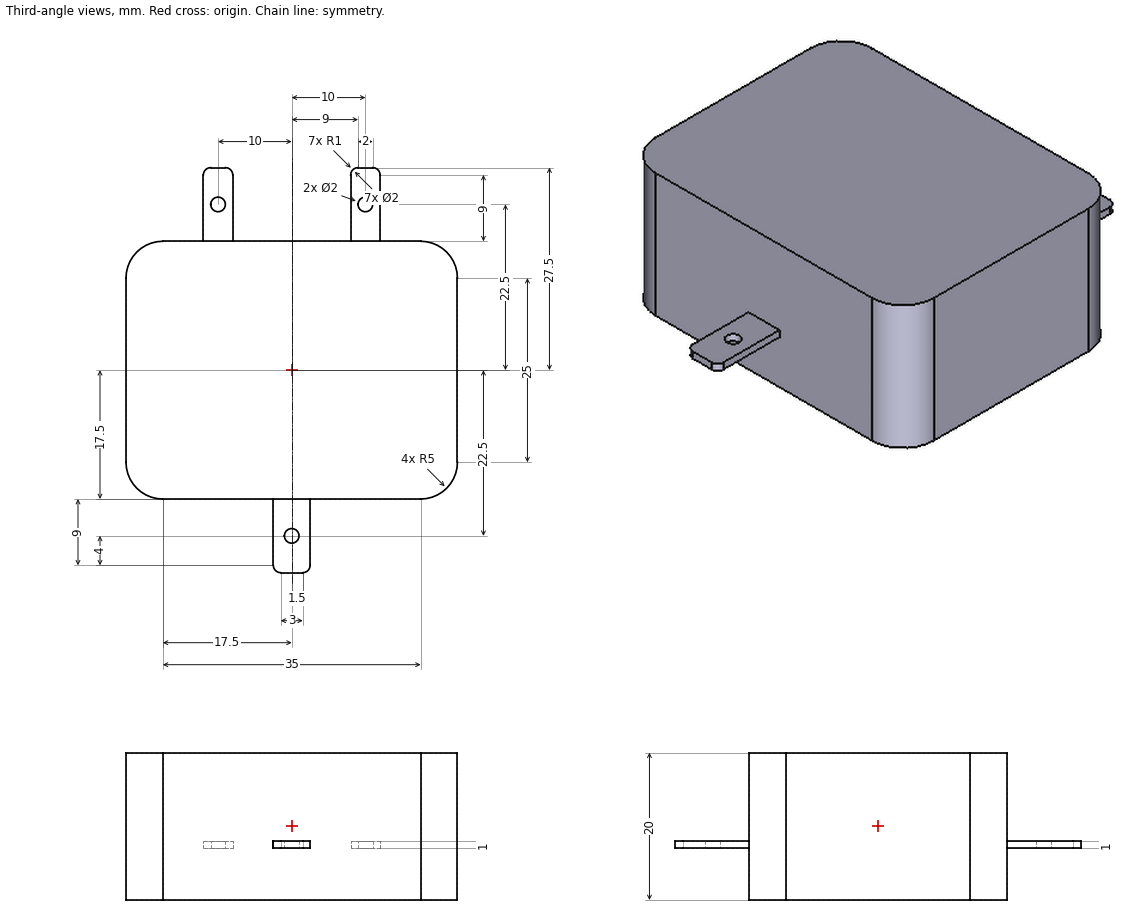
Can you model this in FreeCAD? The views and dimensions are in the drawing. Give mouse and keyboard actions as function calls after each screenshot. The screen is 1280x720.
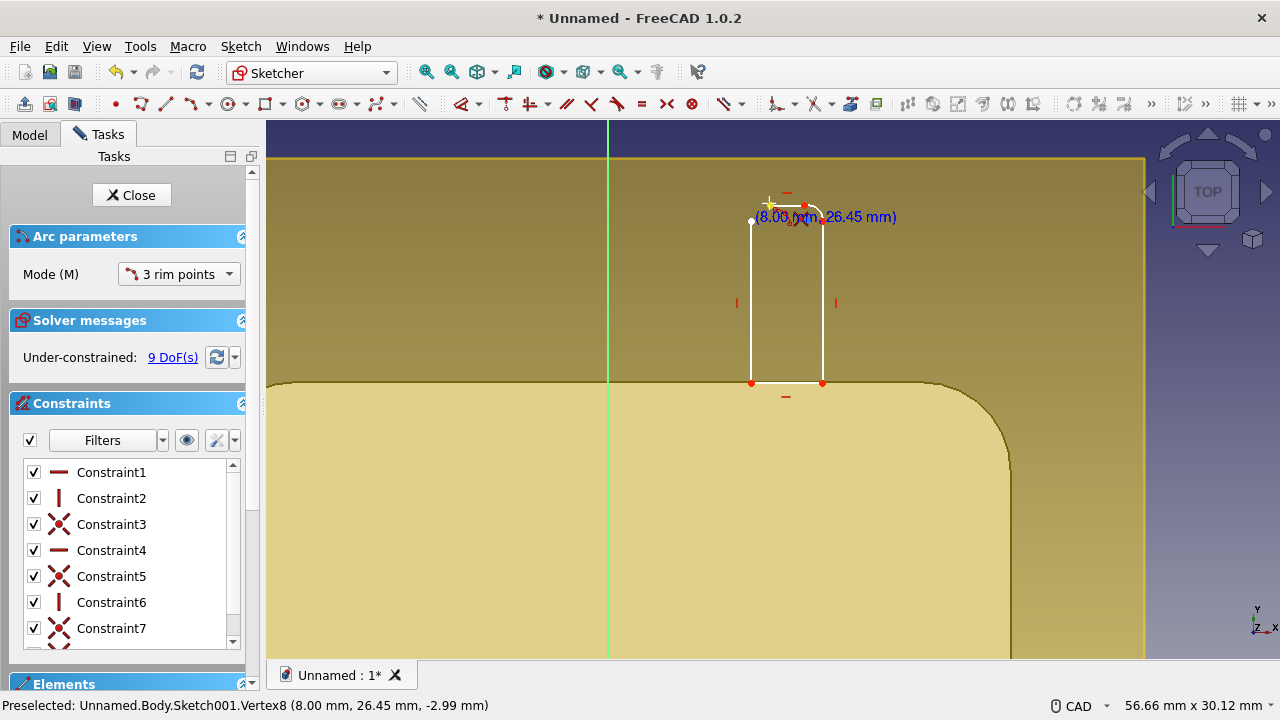
click(771, 206)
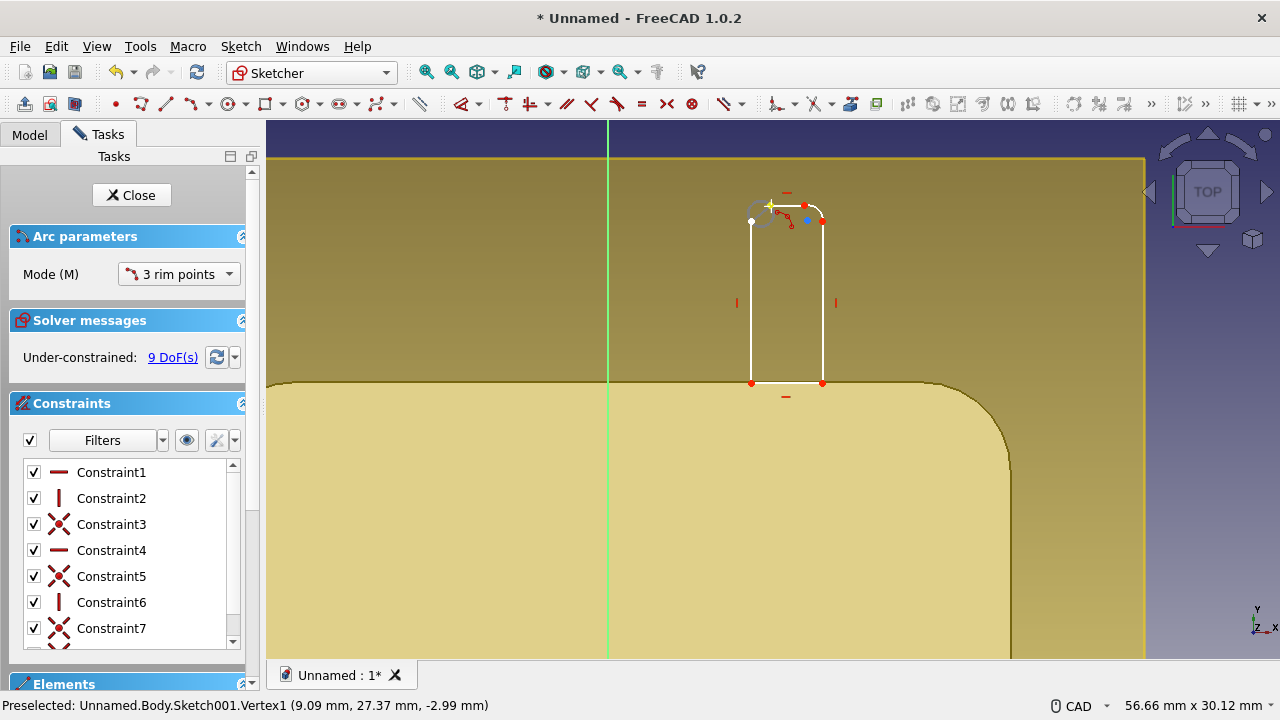
scroll(756, 208, up, 6)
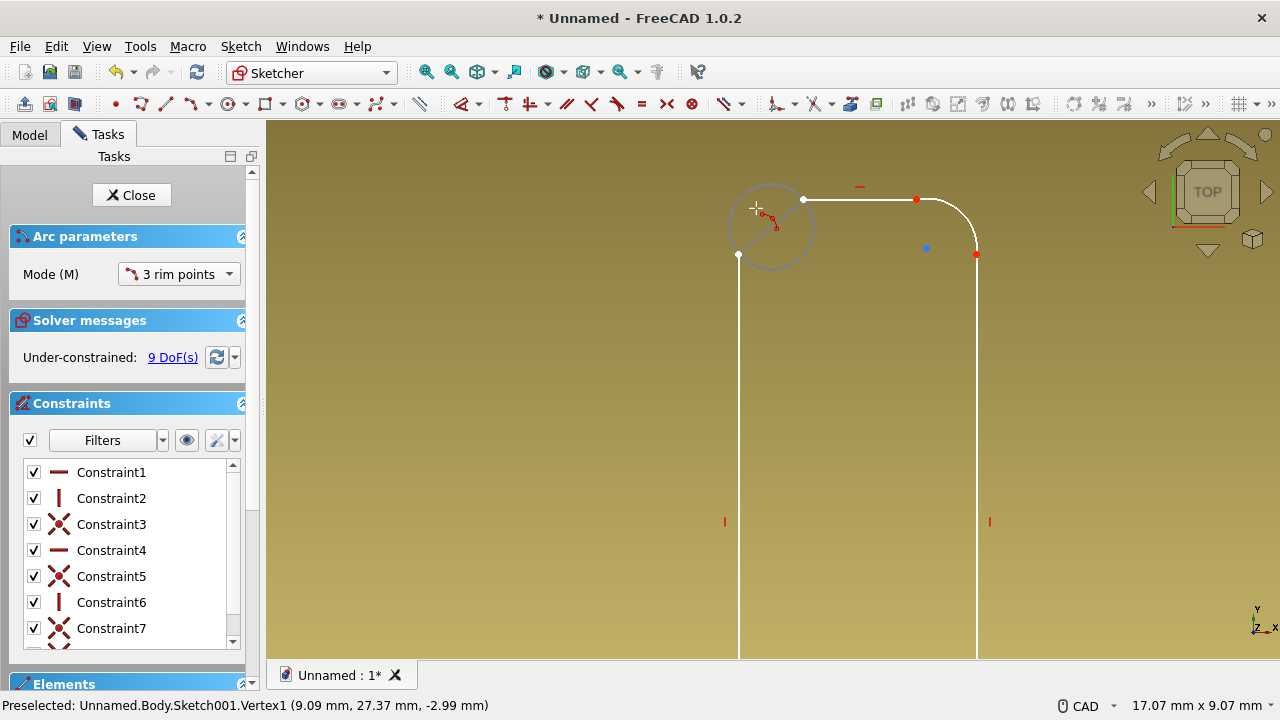
click(756, 209)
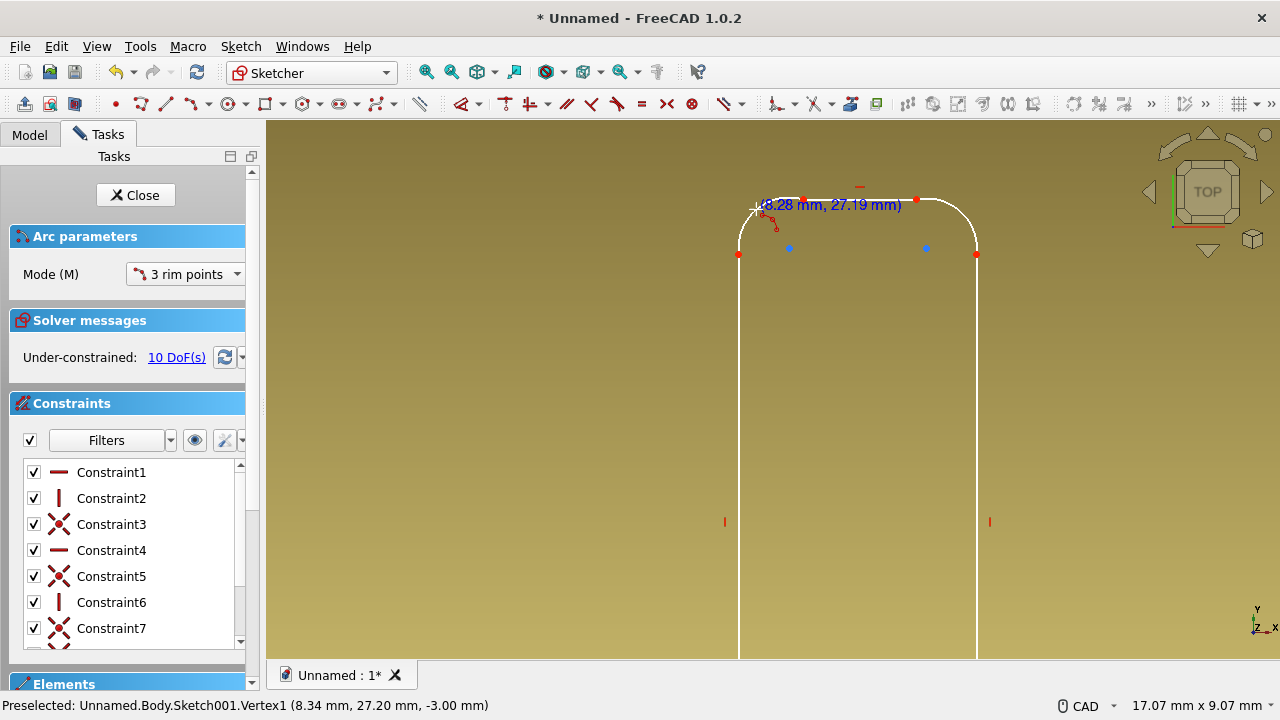
key(g)
key(l)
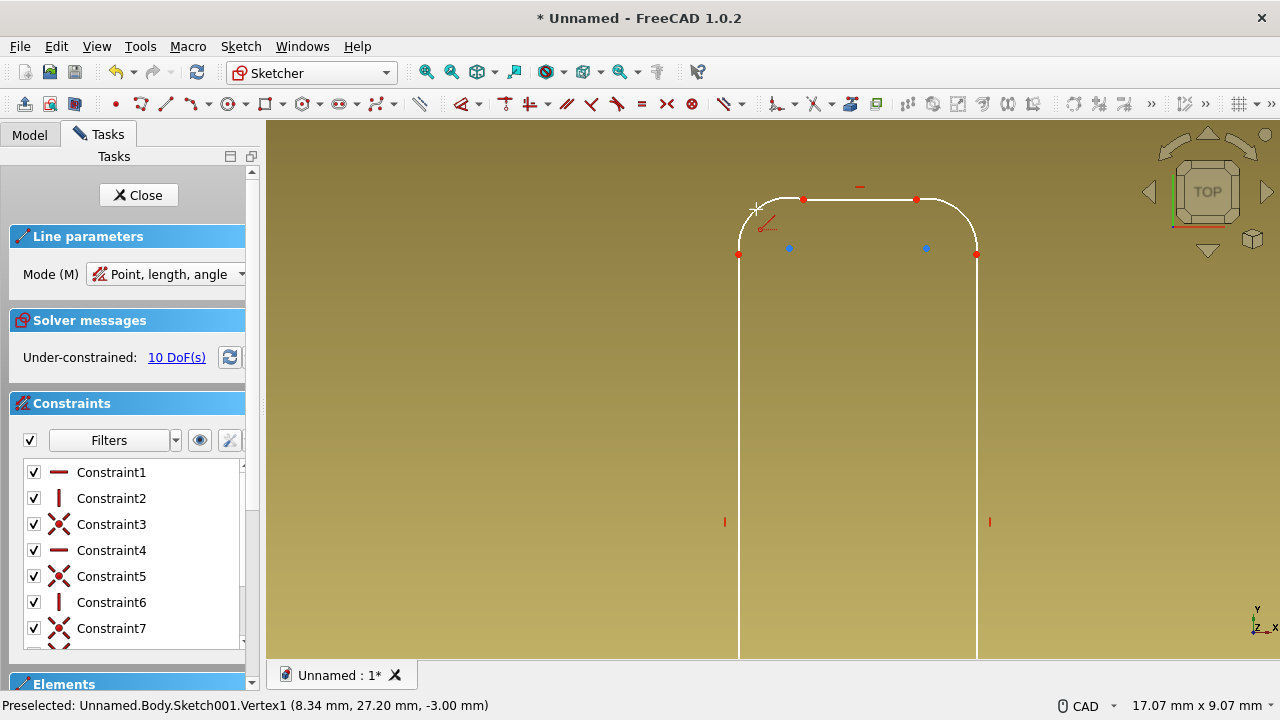
scroll(759, 211, down, 11)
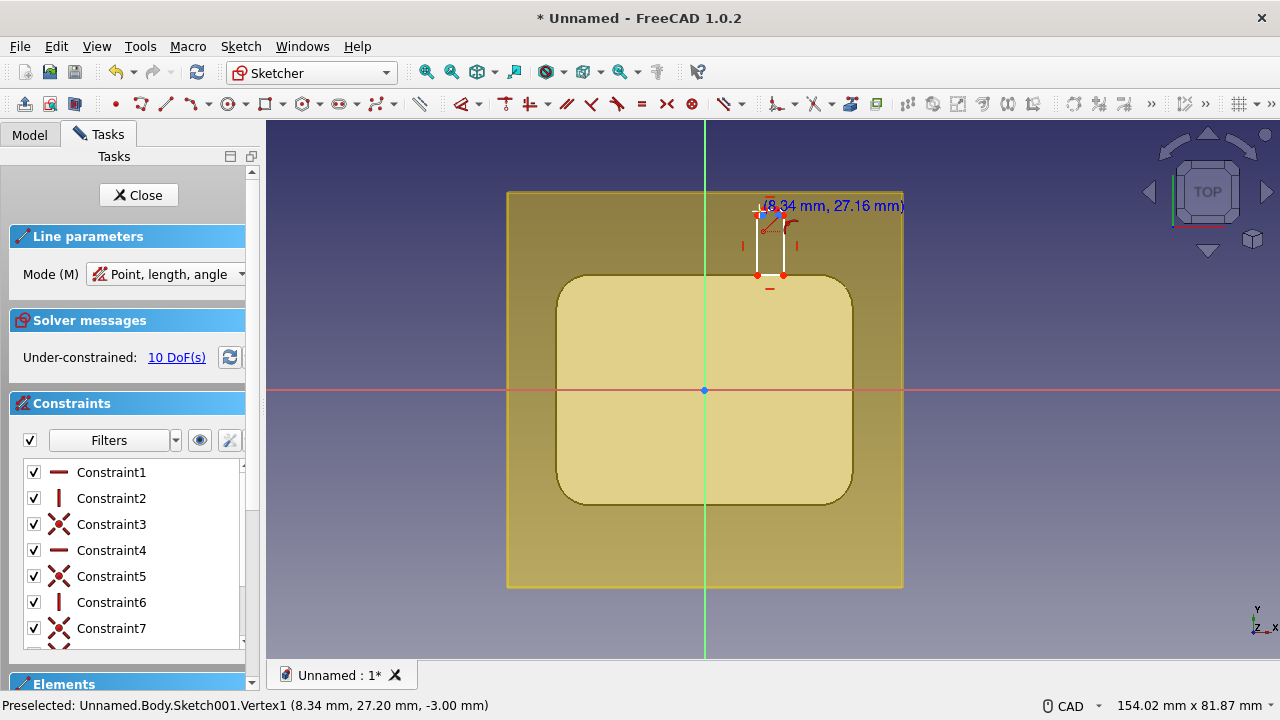
click(632, 209)
click(645, 209)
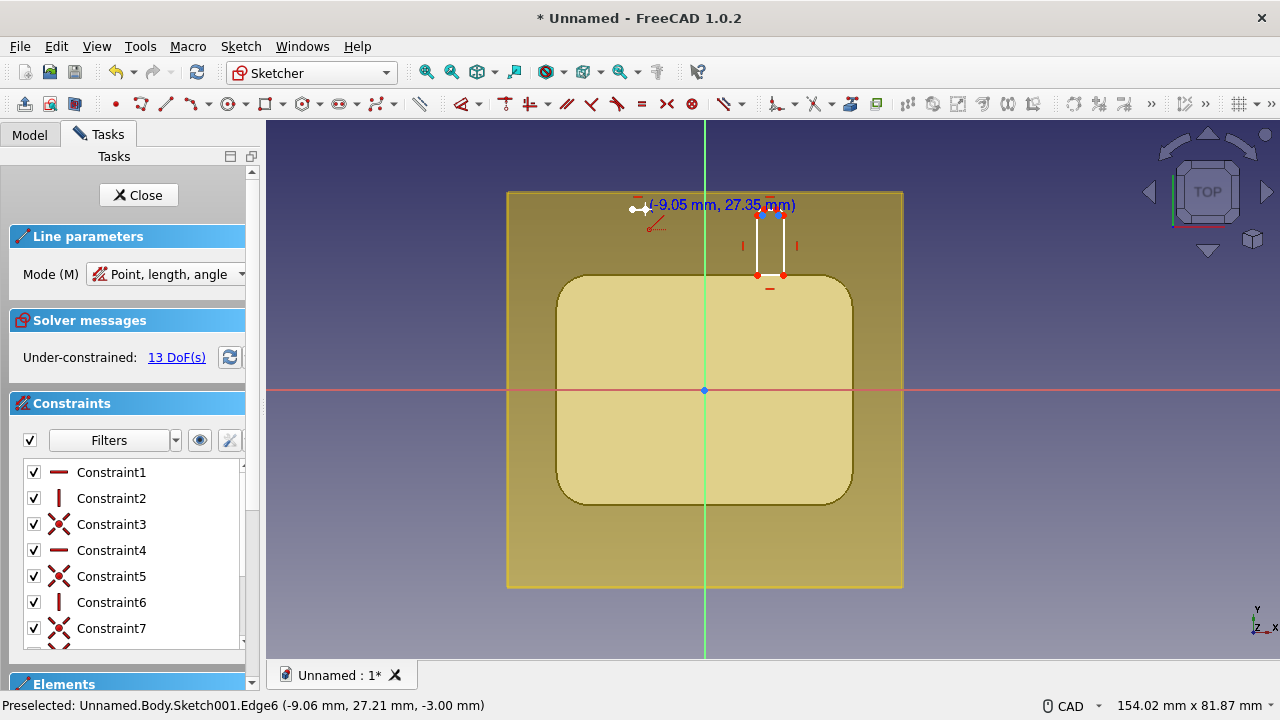
click(141, 104)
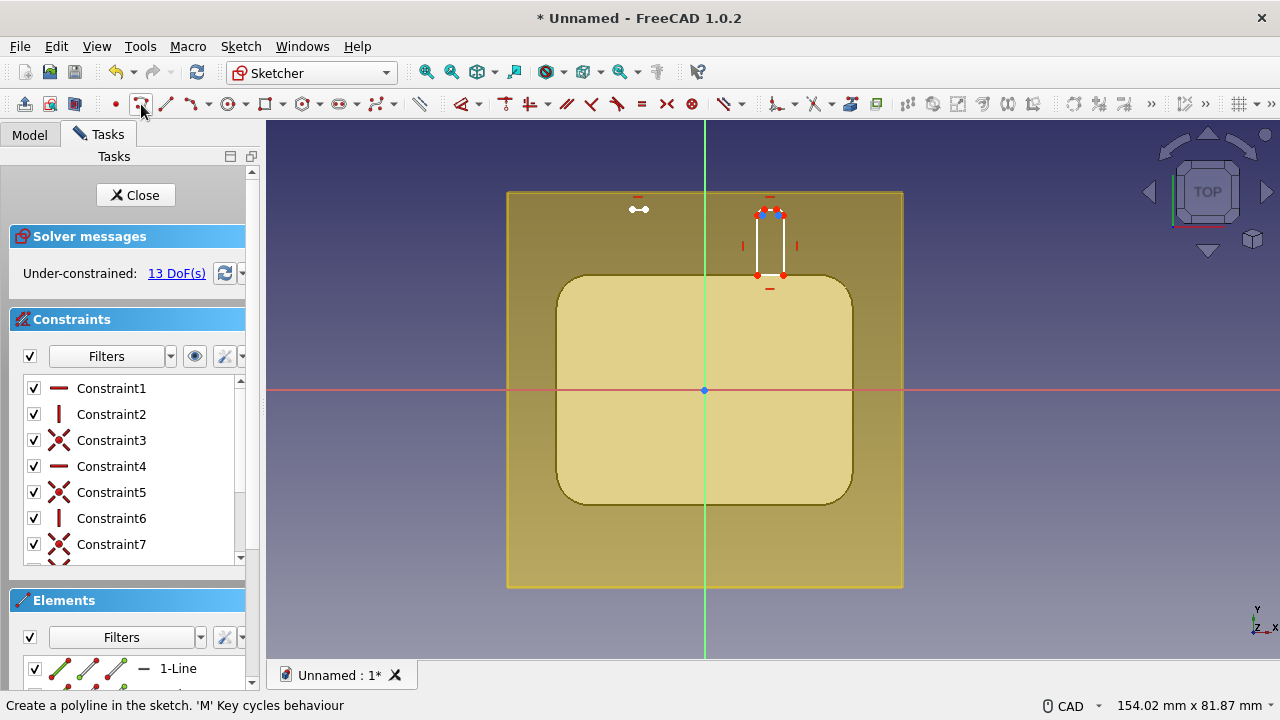
scroll(652, 216, up, 3)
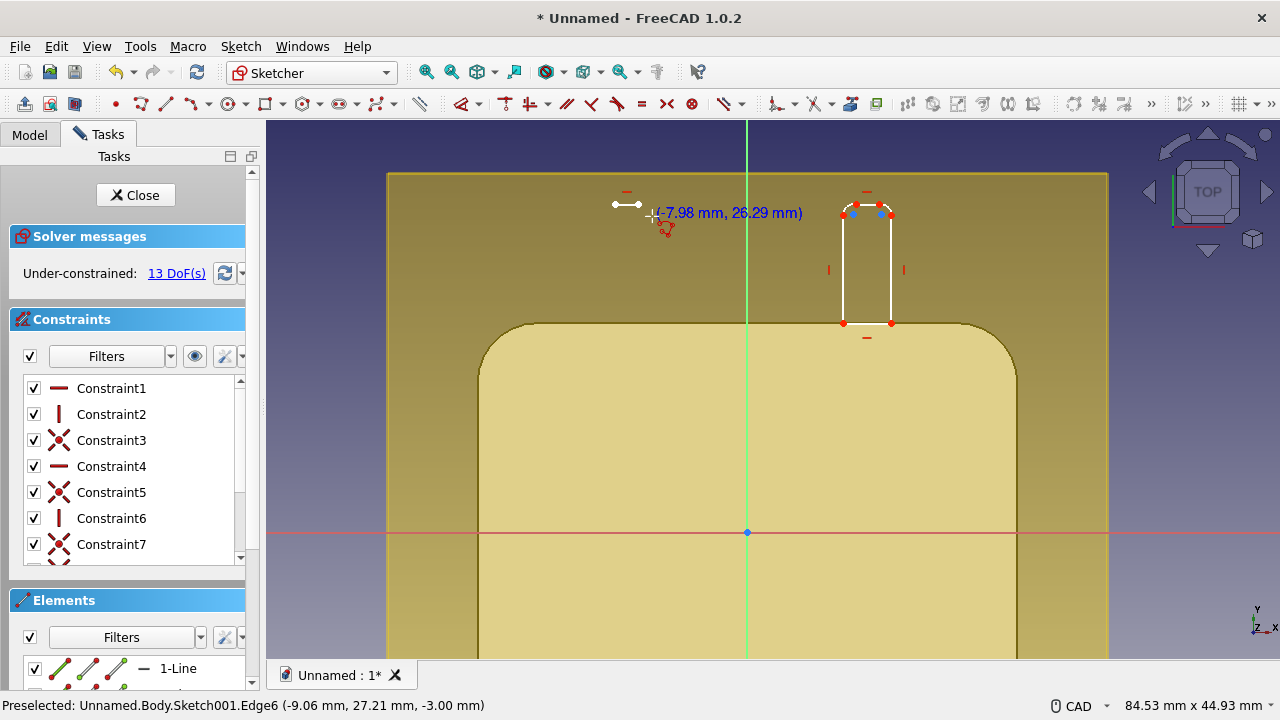
click(651, 215)
click(651, 323)
click(604, 323)
click(604, 215)
right_click(604, 215)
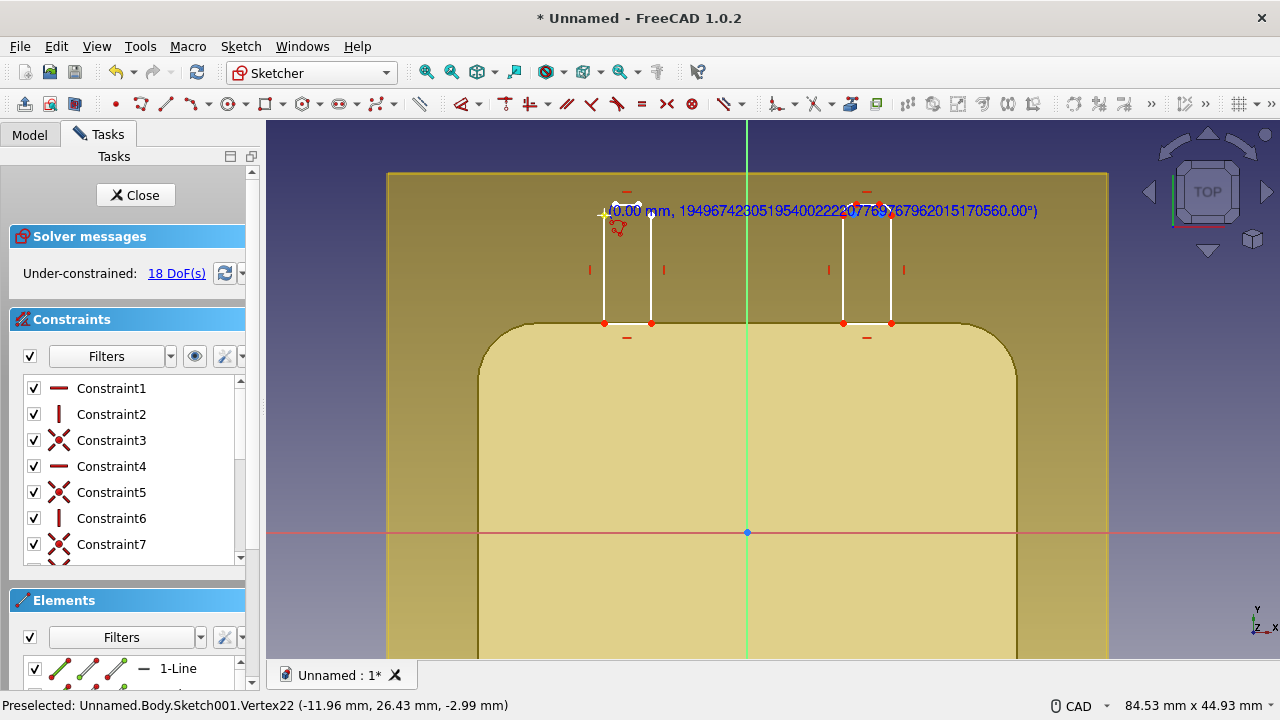
click(190, 104)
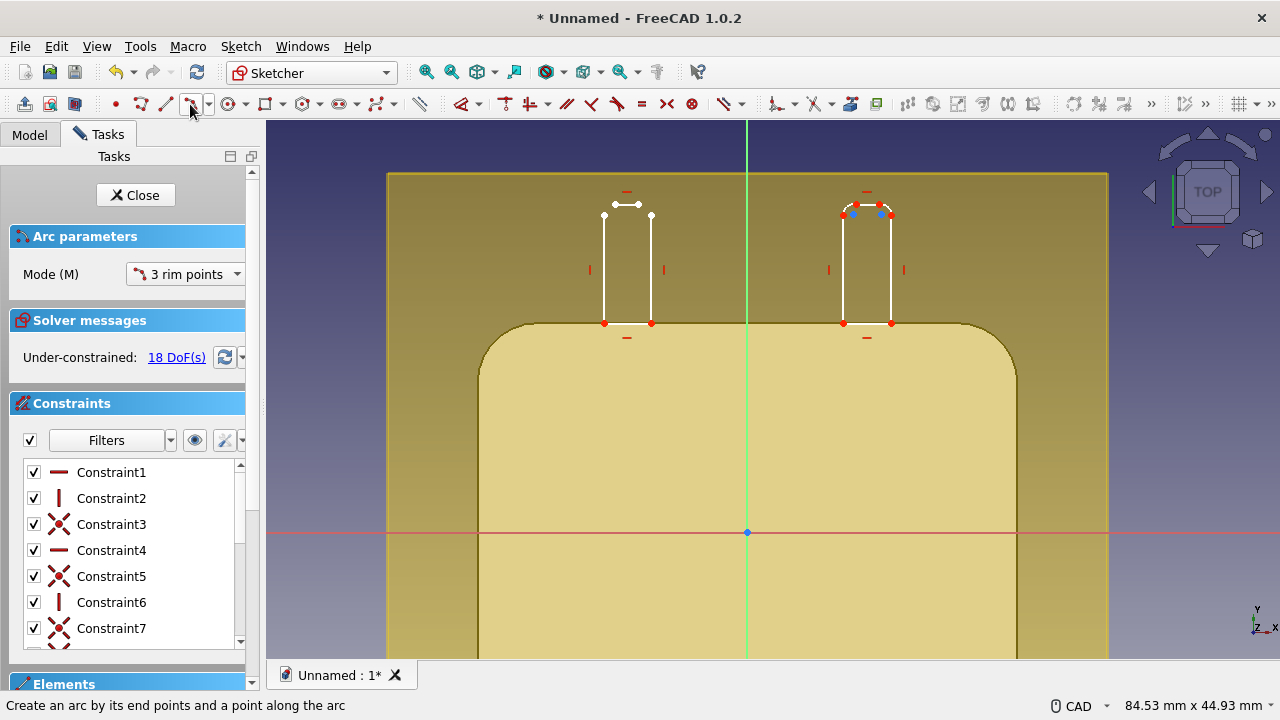
scroll(639, 203, up, 2)